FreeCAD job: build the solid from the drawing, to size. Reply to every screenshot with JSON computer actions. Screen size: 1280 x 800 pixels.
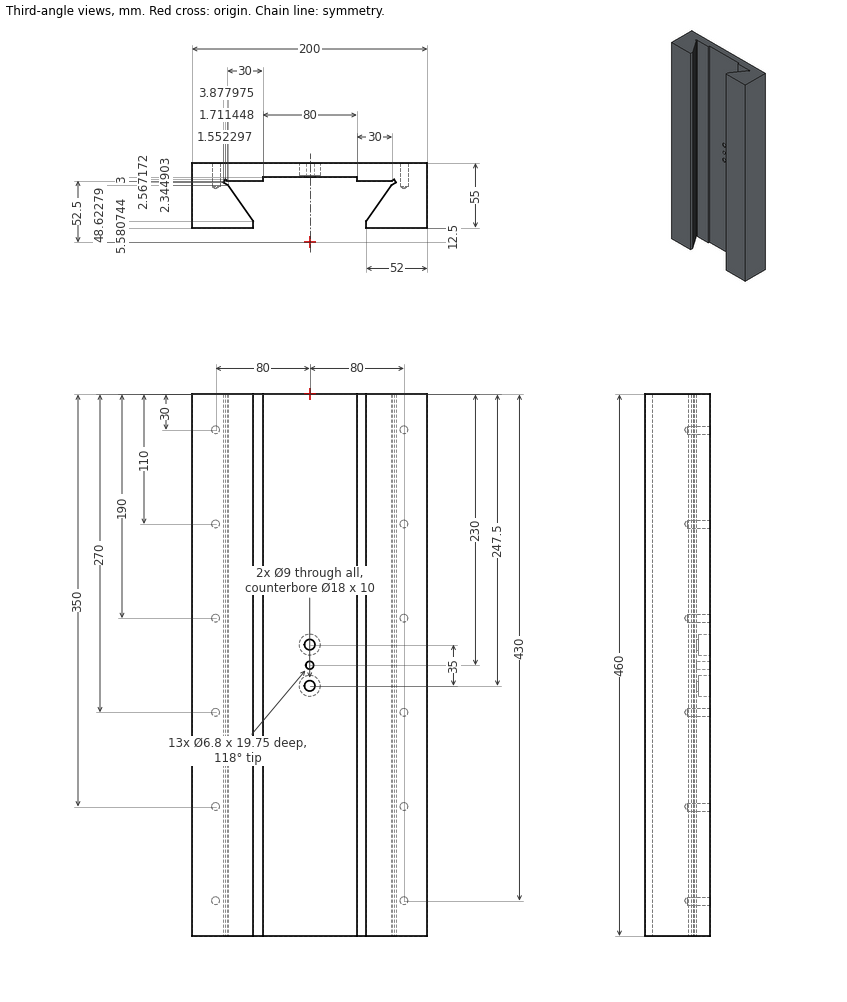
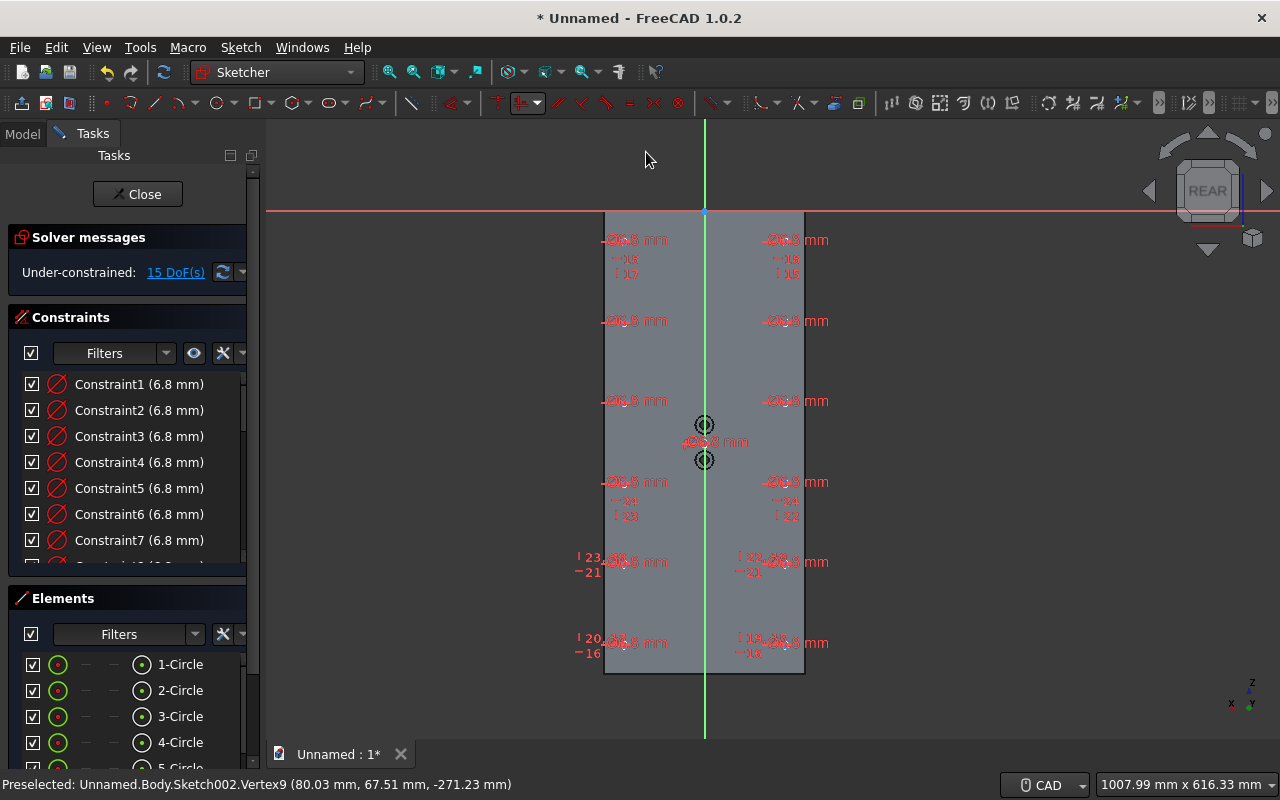
{"action": "left_click", "coordinate": [785, 484]}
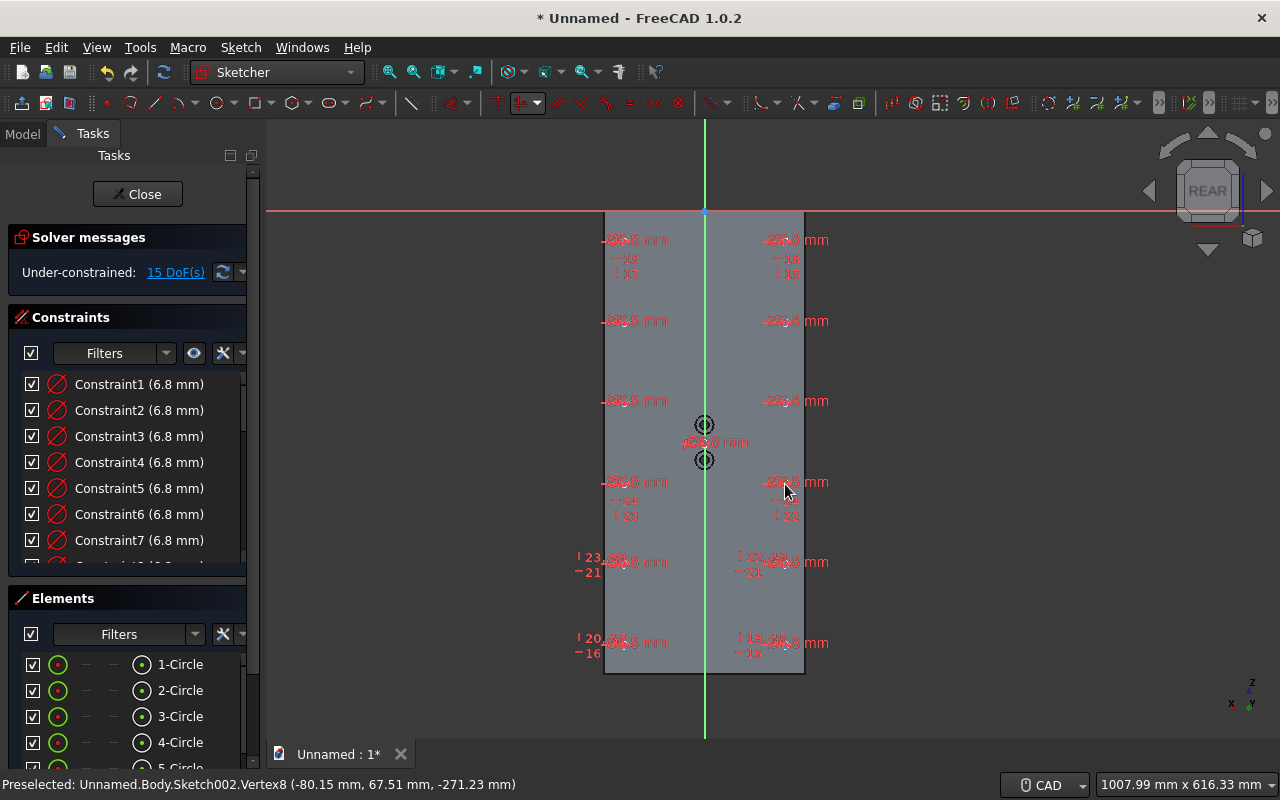
{"action": "left_click", "coordinate": [785, 403]}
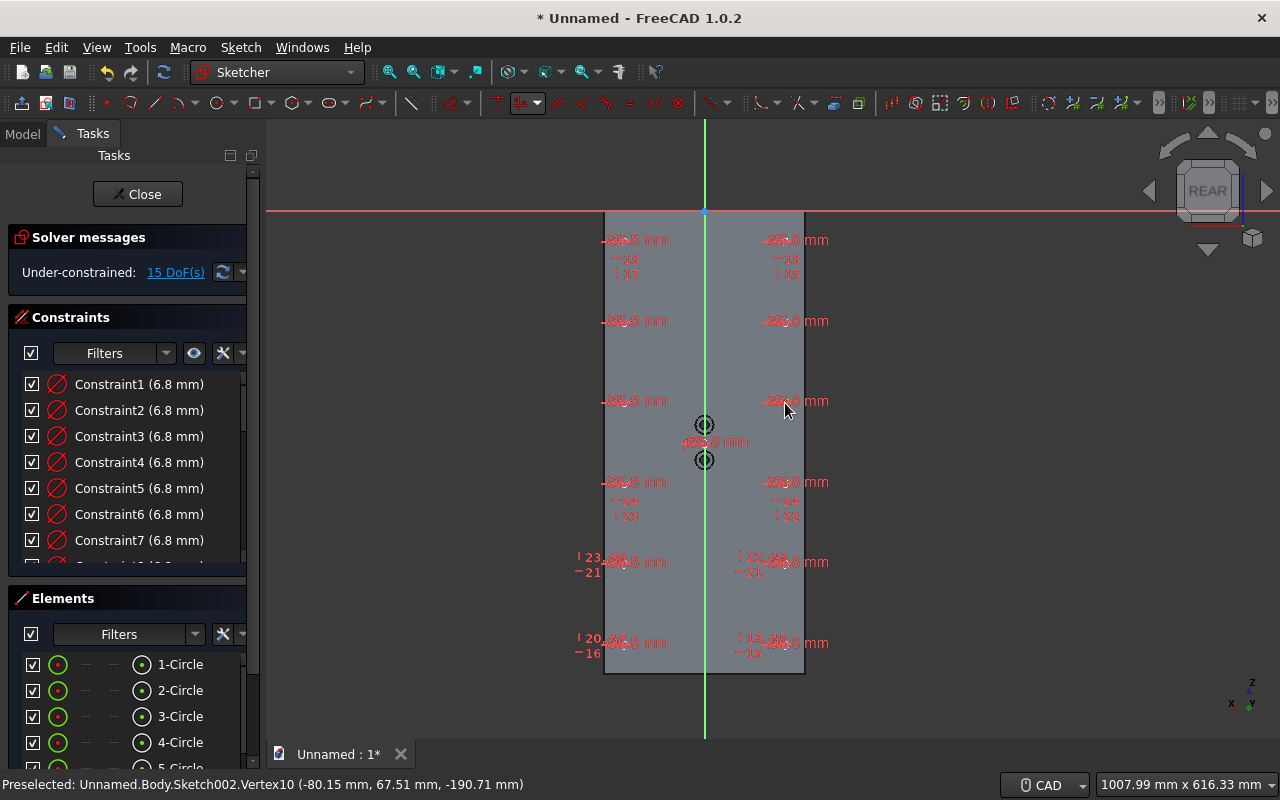
{"action": "left_click", "coordinate": [540, 104]}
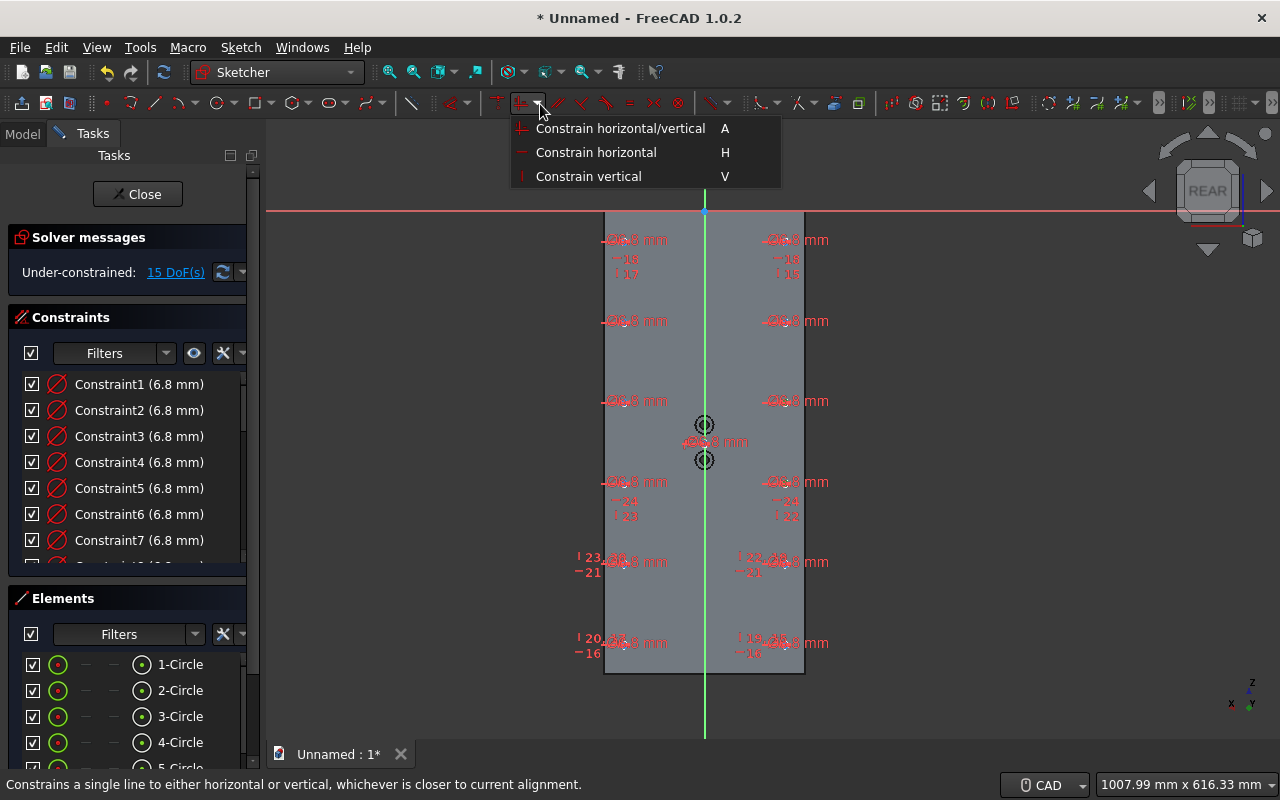
{"action": "left_click", "coordinate": [646, 176]}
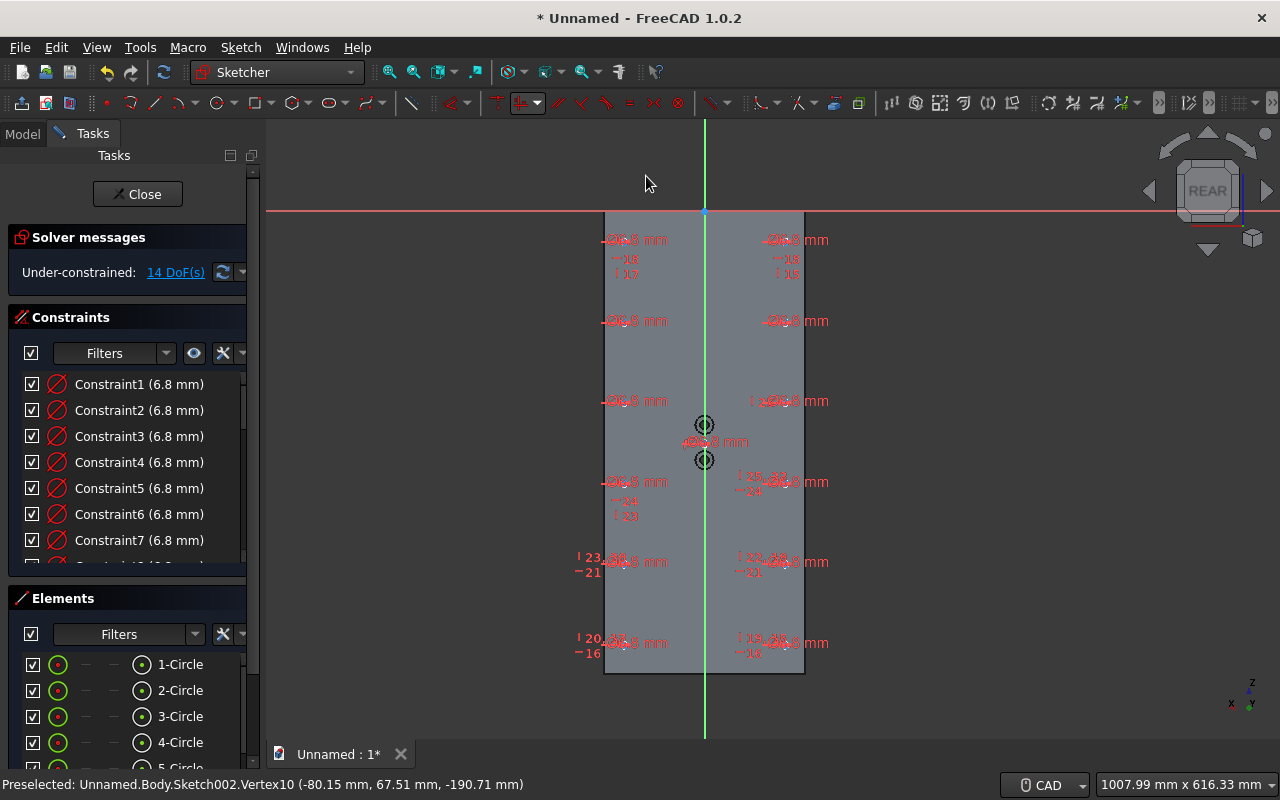
{"action": "left_click", "coordinate": [624, 484]}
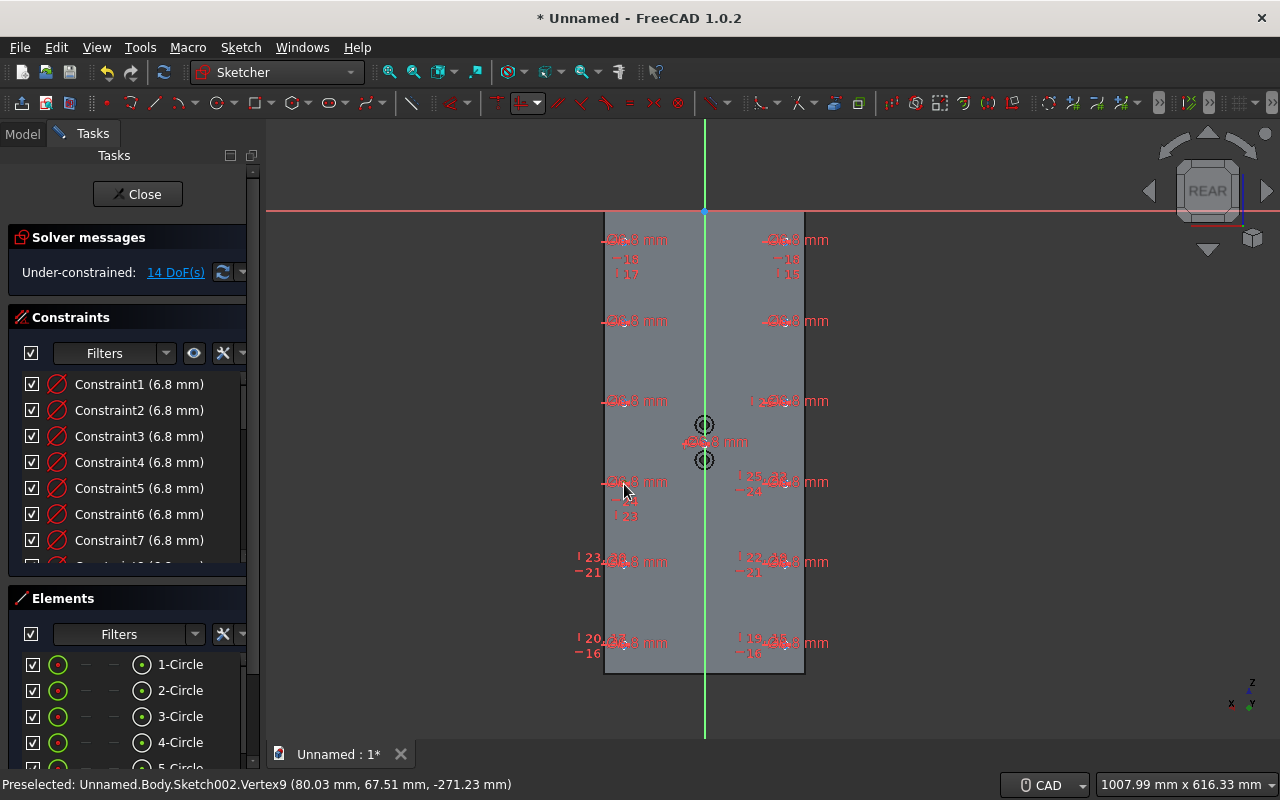
{"action": "left_click", "coordinate": [624, 403]}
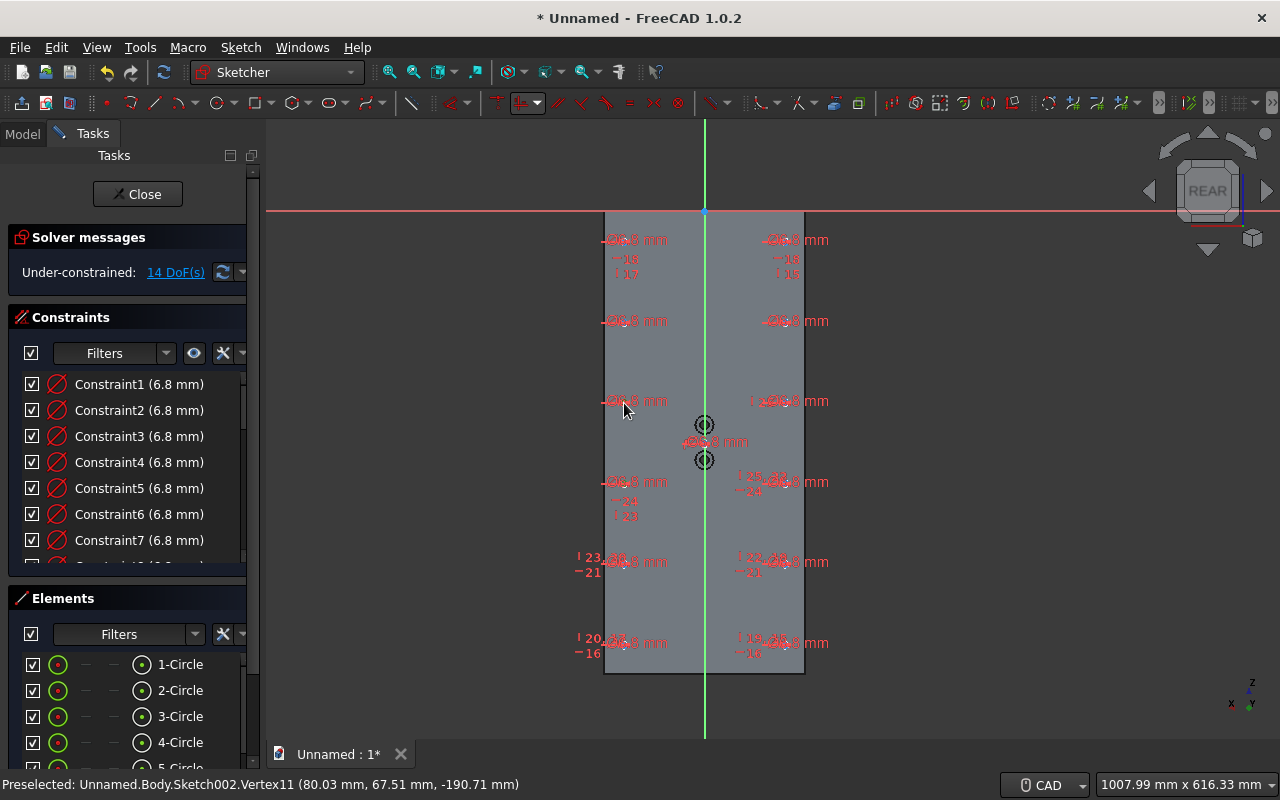
{"action": "left_click", "coordinate": [540, 104]}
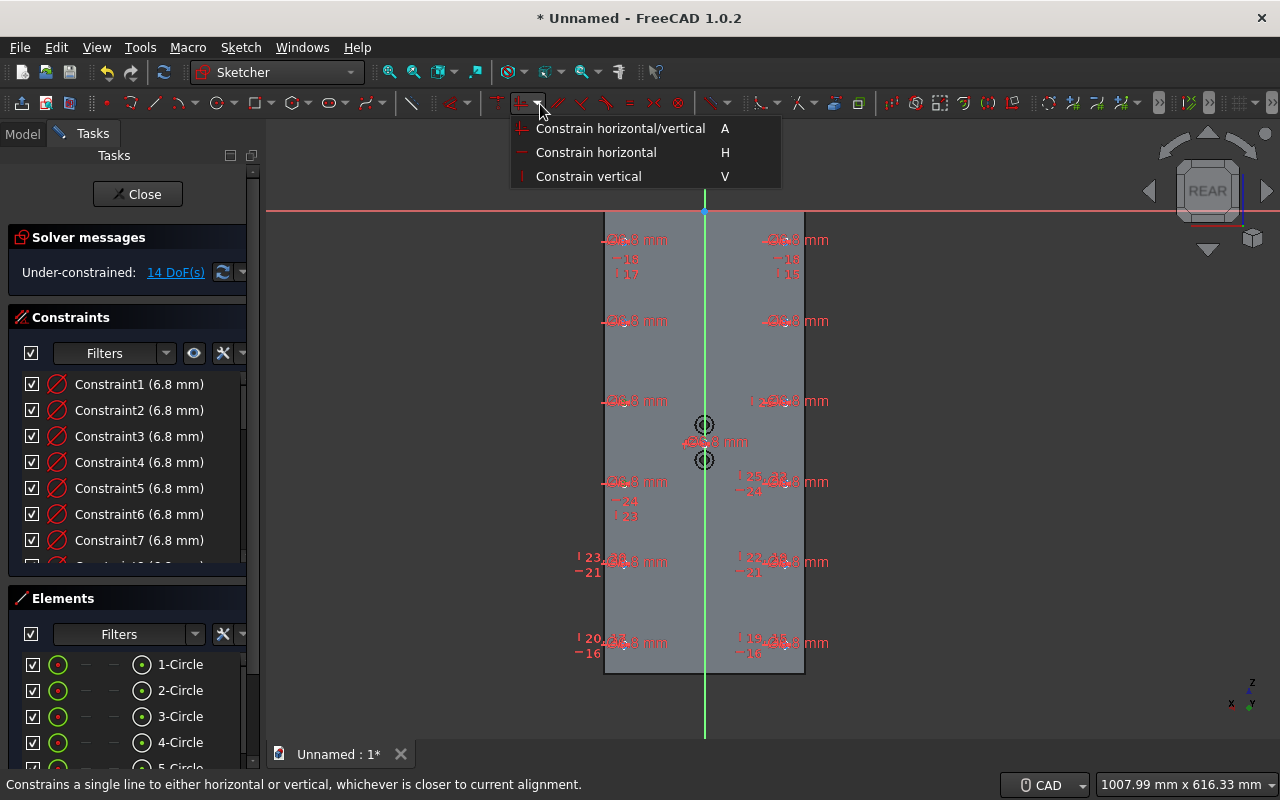
{"action": "left_click", "coordinate": [646, 176]}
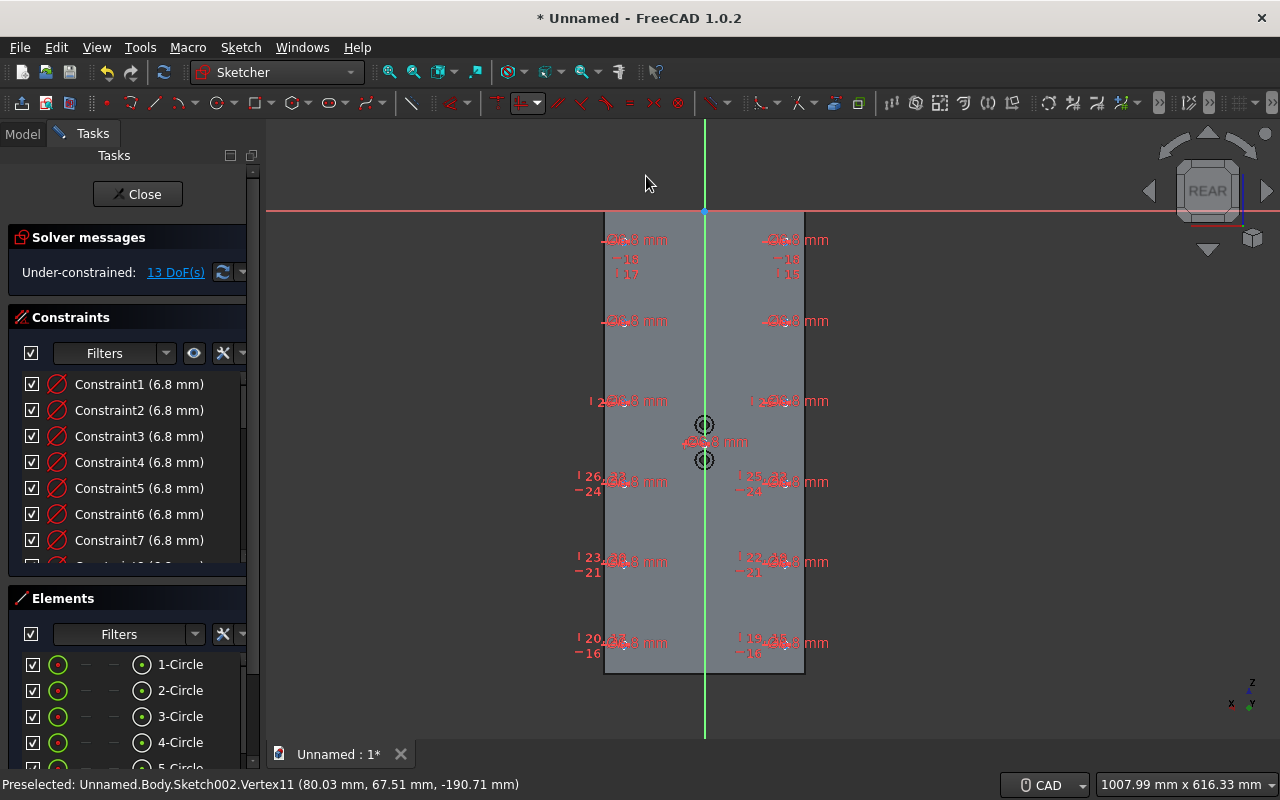
{"action": "left_click", "coordinate": [785, 403]}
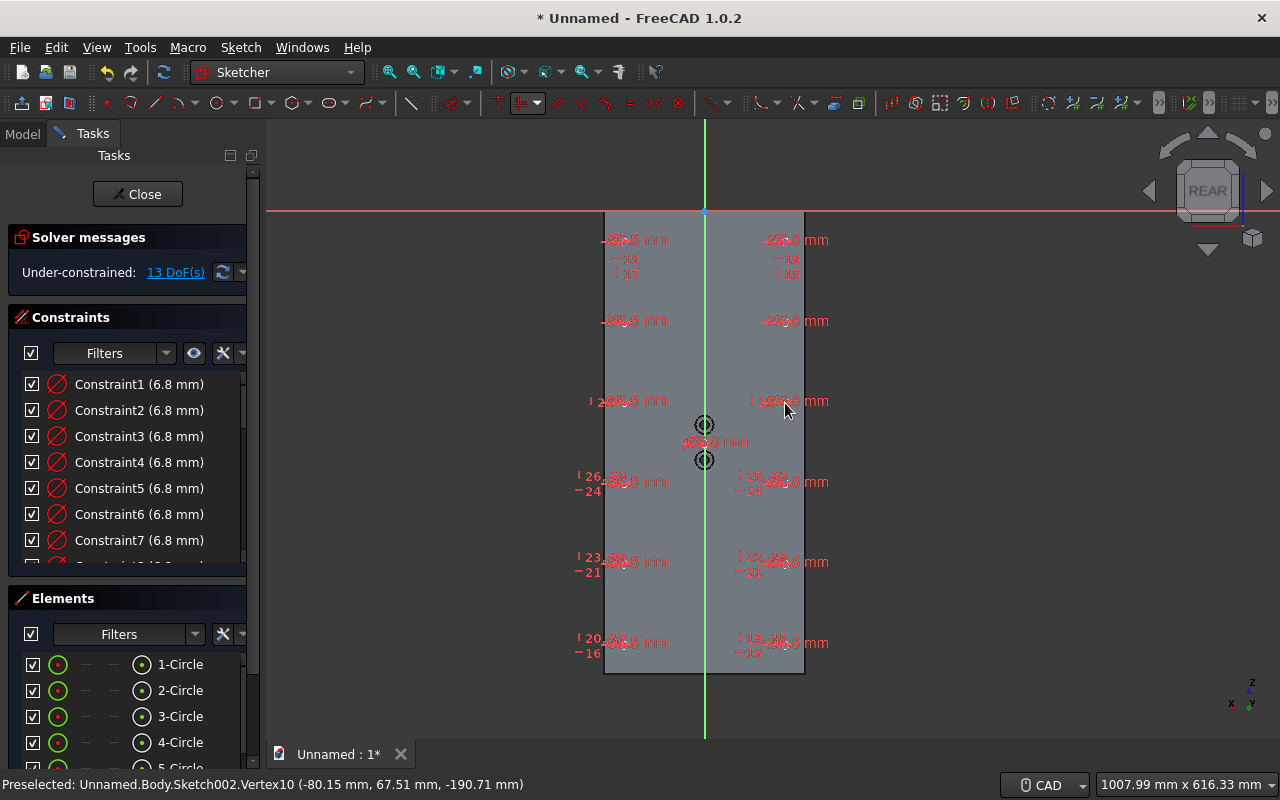
{"action": "left_click", "coordinate": [624, 403]}